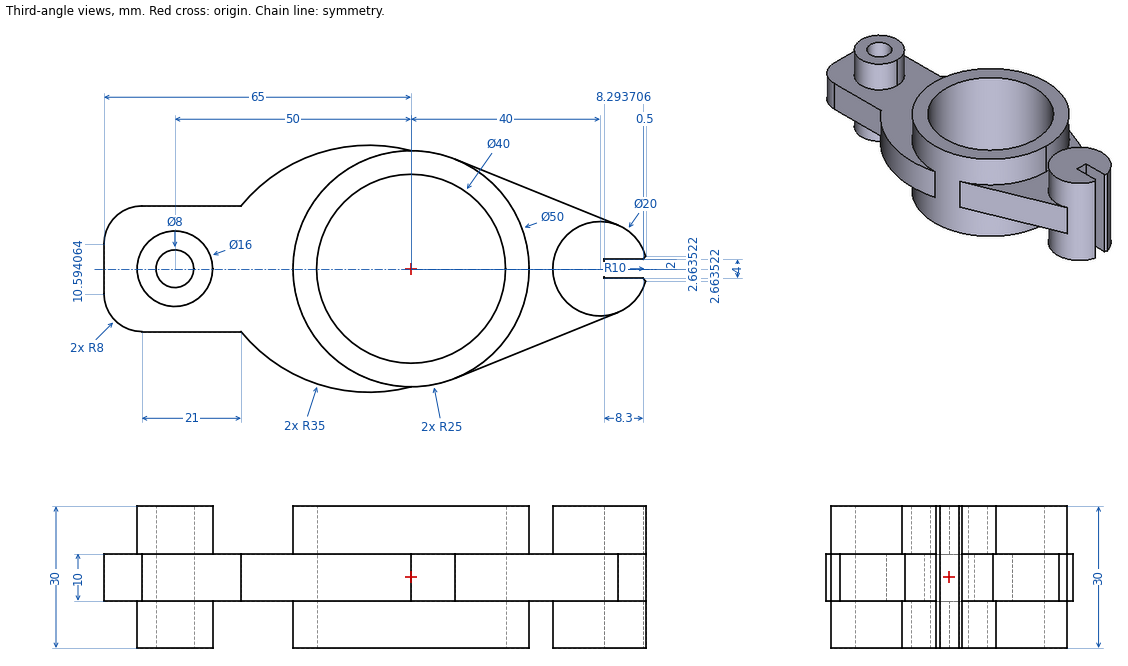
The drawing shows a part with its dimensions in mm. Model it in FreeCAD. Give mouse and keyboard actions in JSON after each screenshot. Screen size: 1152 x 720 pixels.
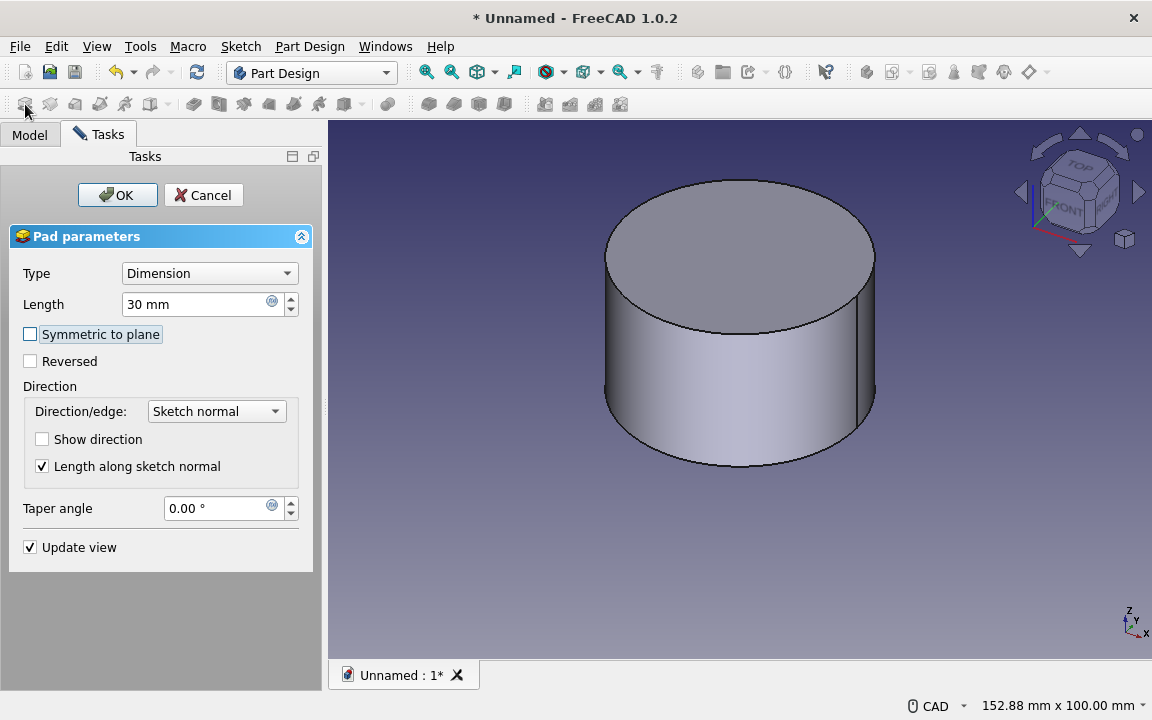
{"action": "left_click", "coordinate": [31, 334]}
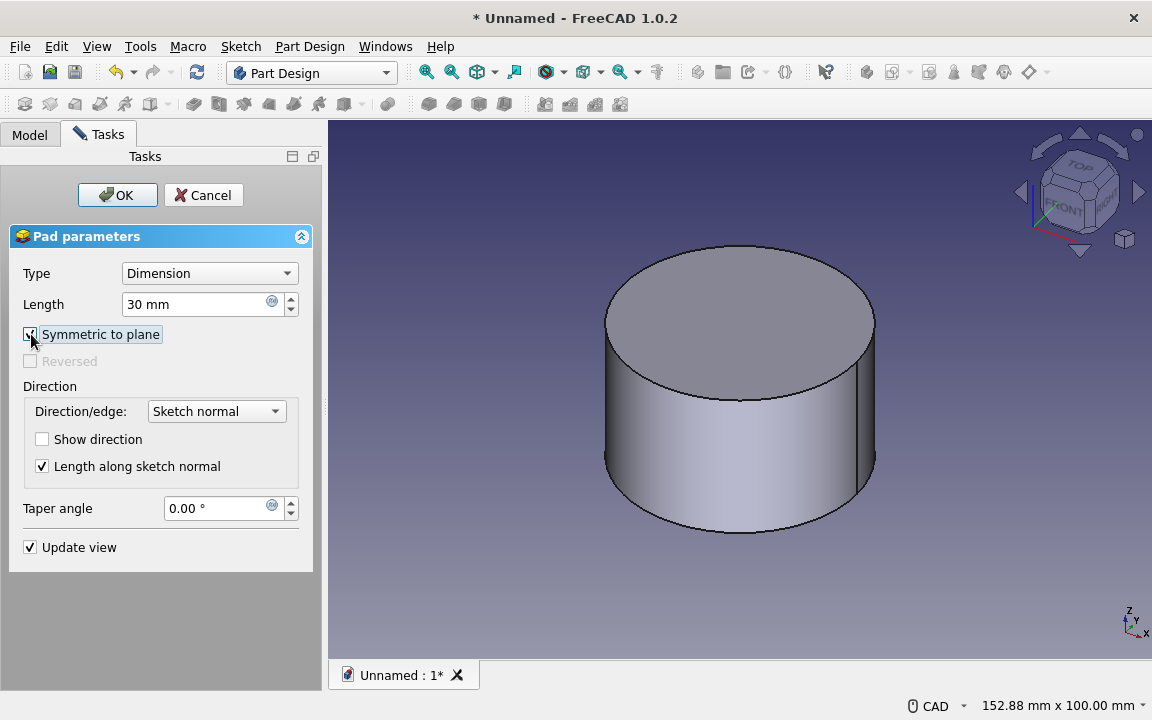
{"action": "left_click", "coordinate": [118, 195]}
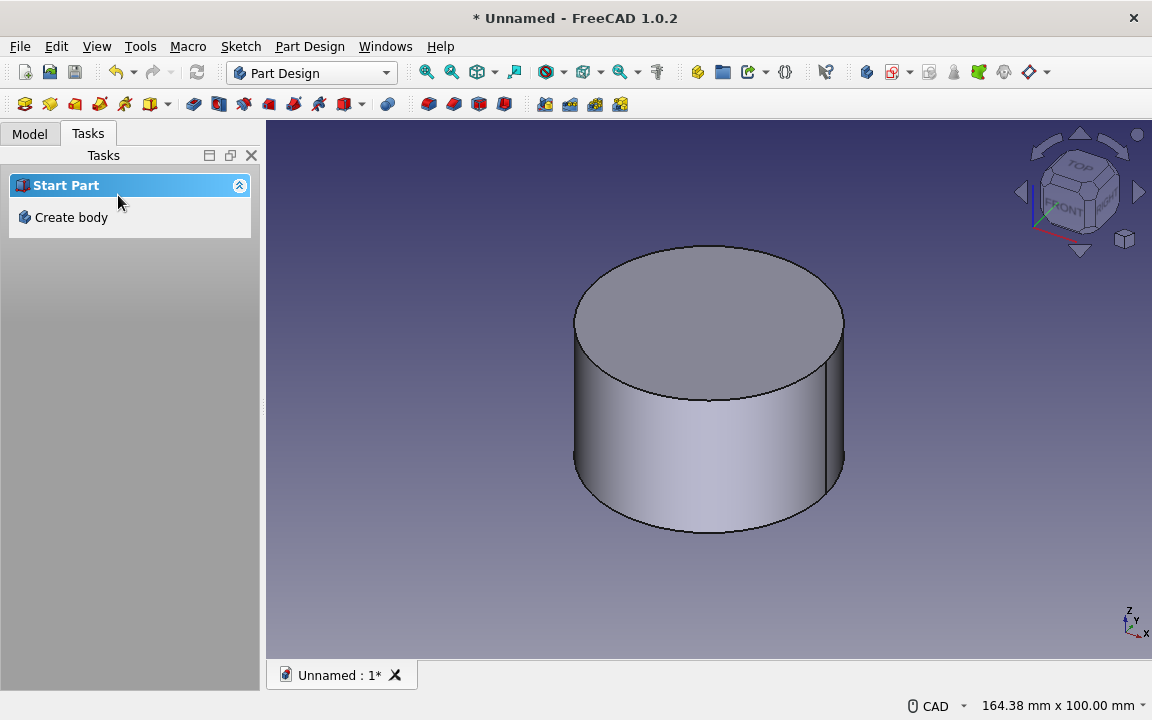
{"action": "left_click", "coordinate": [867, 72]}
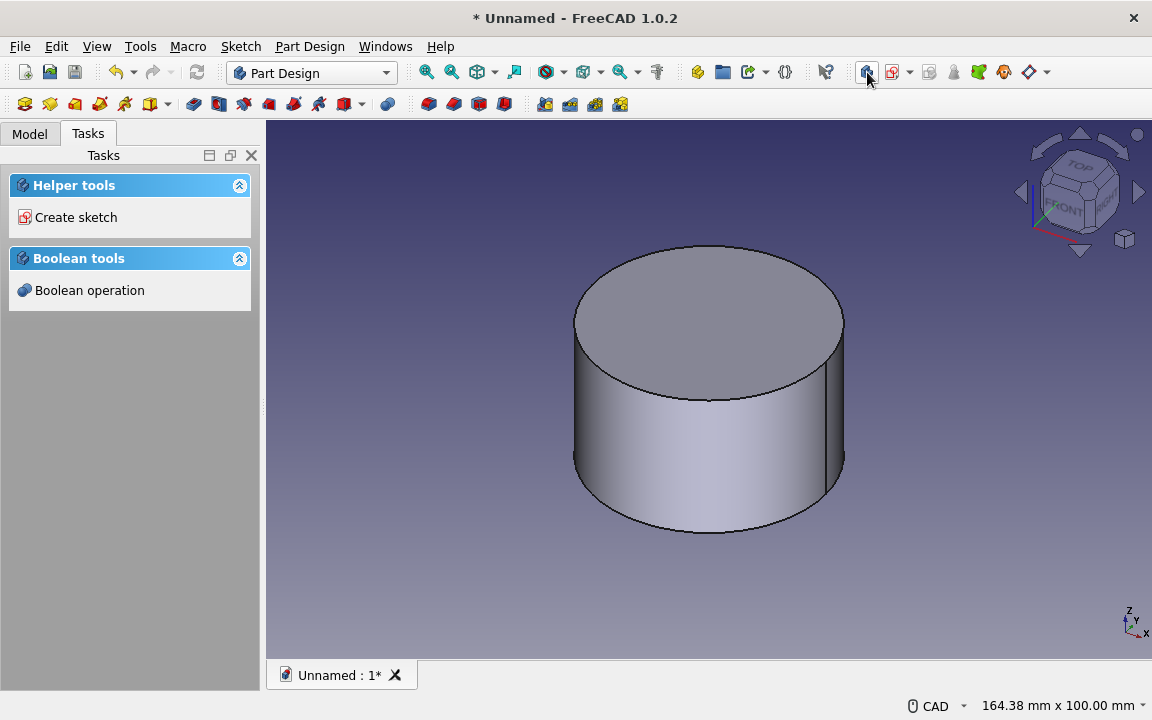
{"action": "left_click", "coordinate": [306, 619]}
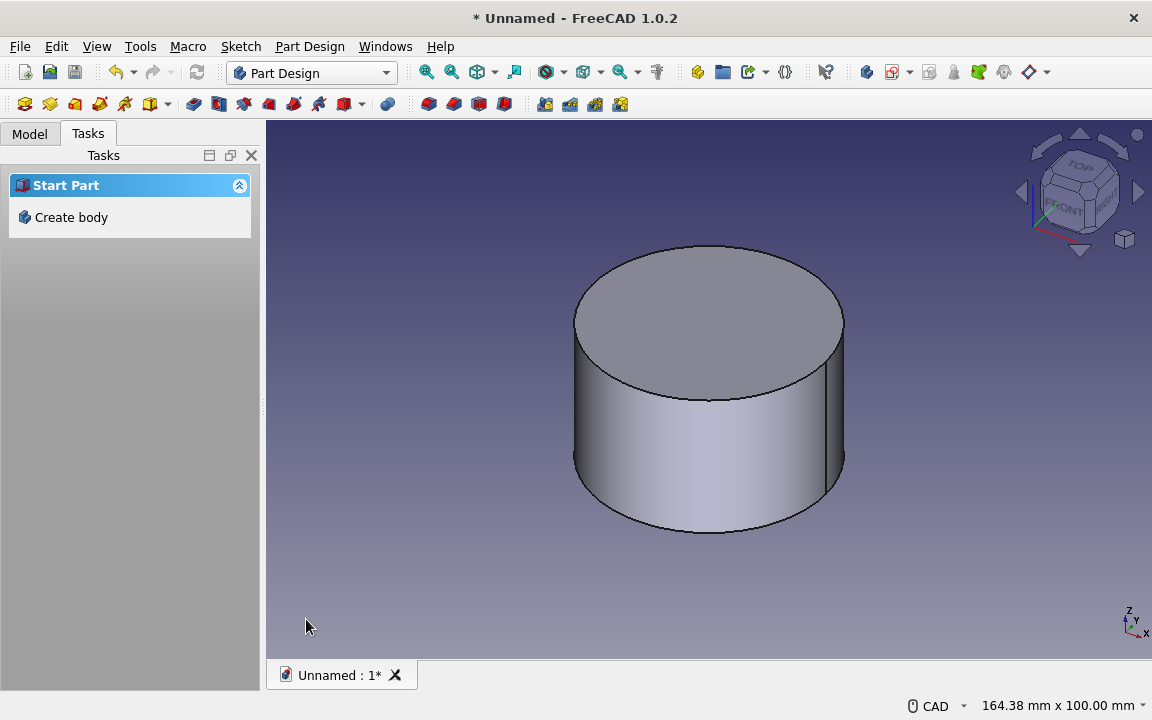
{"action": "left_click", "coordinate": [892, 72]}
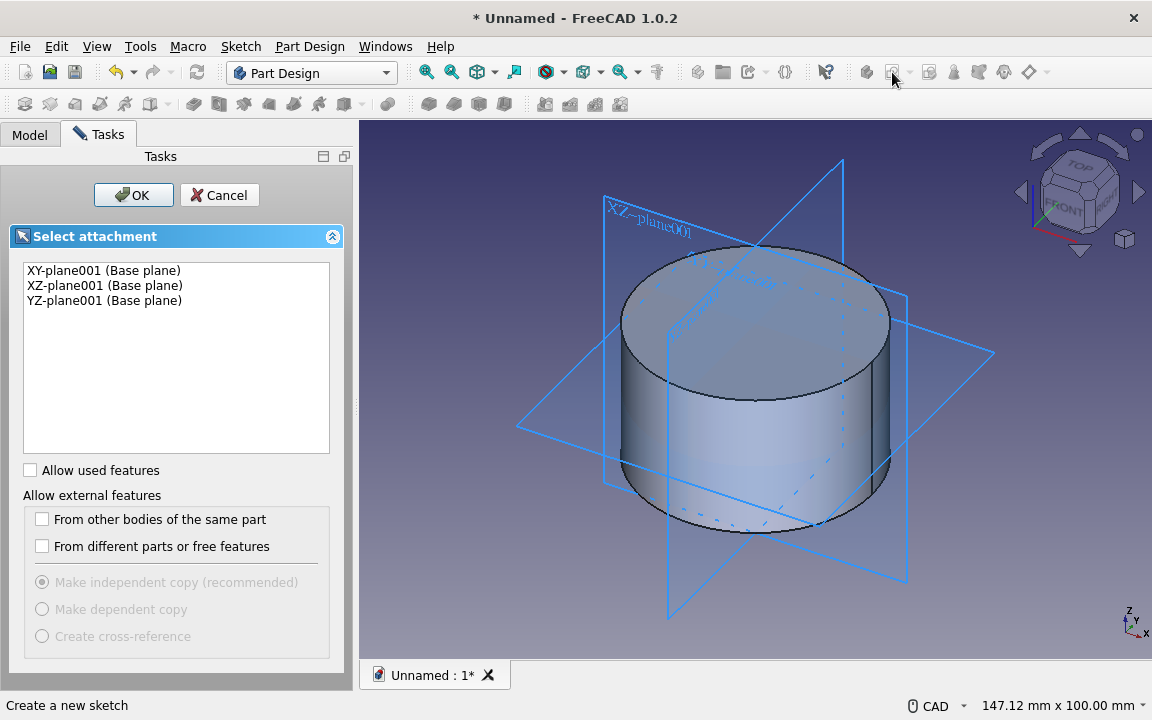
{"action": "left_click", "coordinate": [84, 270]}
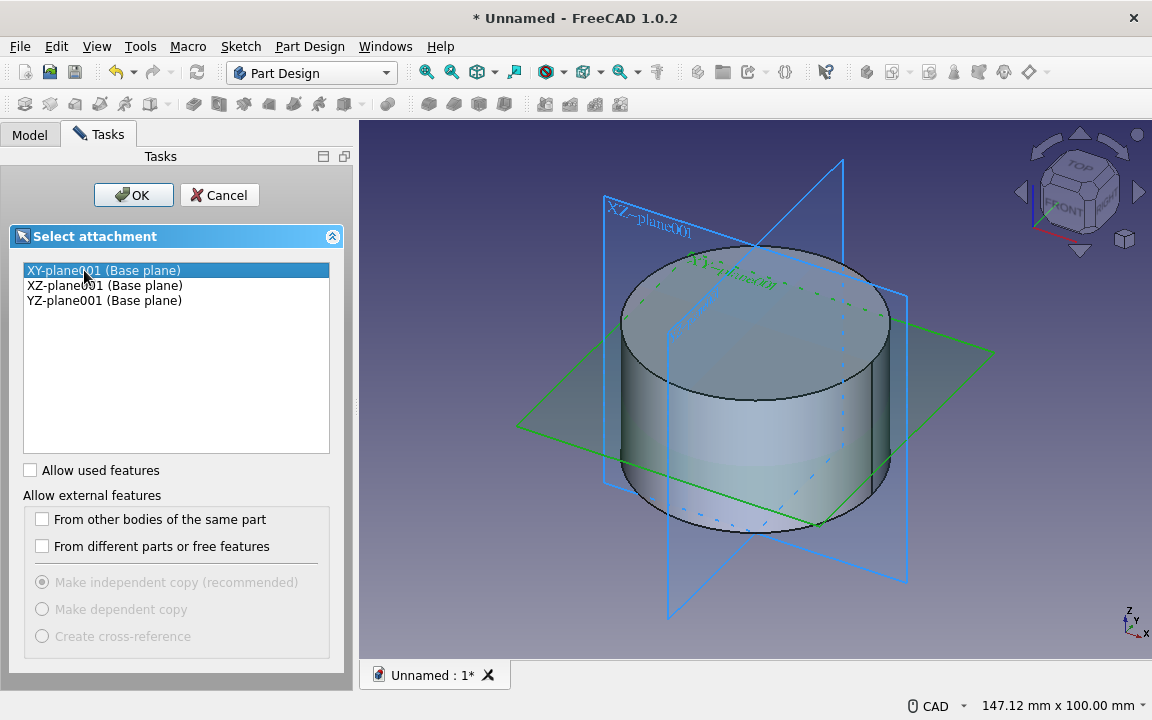
{"action": "left_click", "coordinate": [134, 195]}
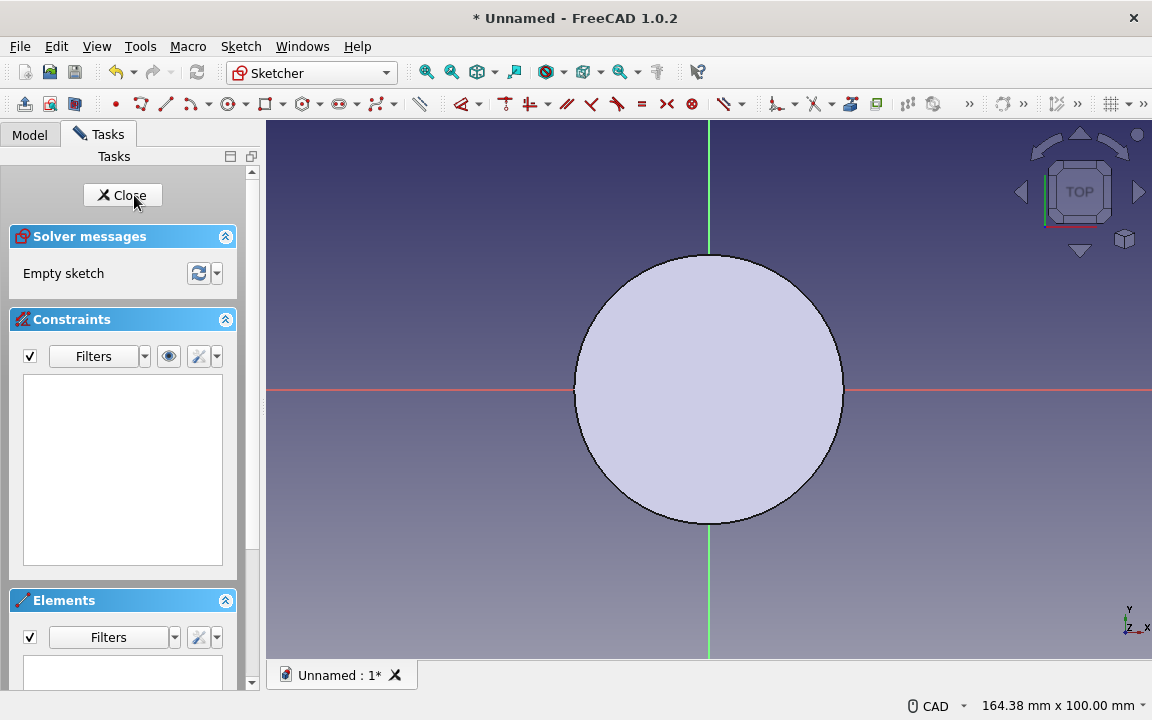
{"action": "scroll", "coordinate": [374, 390], "scroll_direction": "up", "scroll_amount": 7}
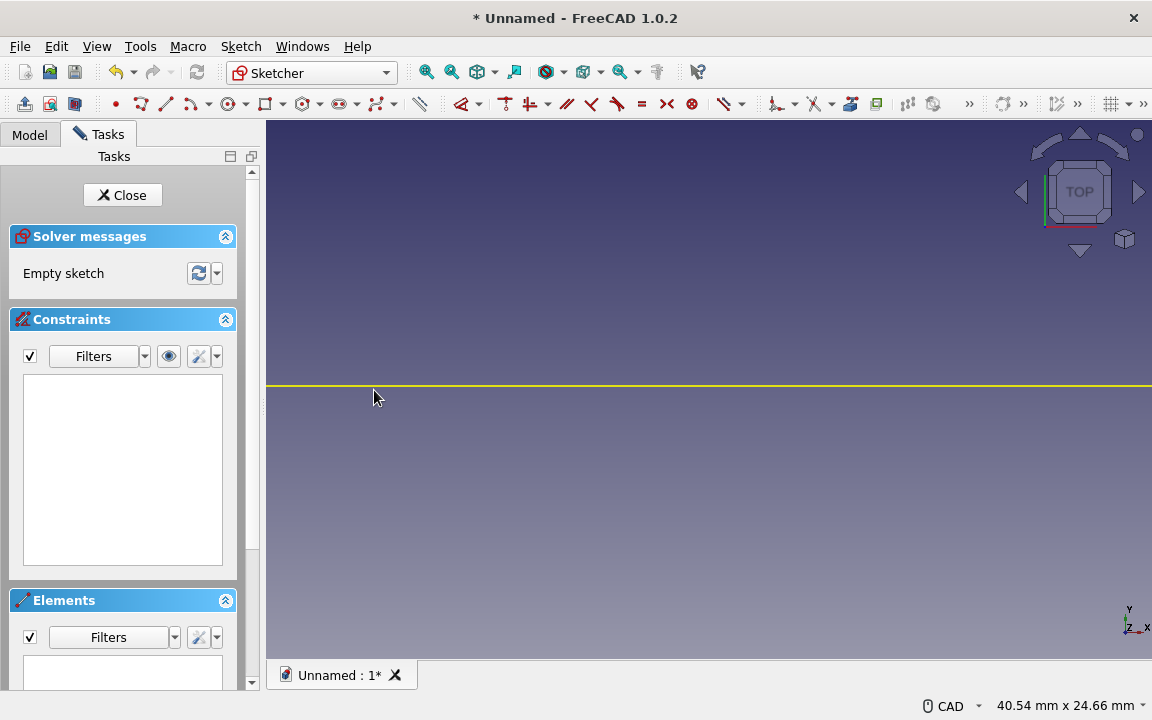
{"action": "left_click", "coordinate": [228, 104]}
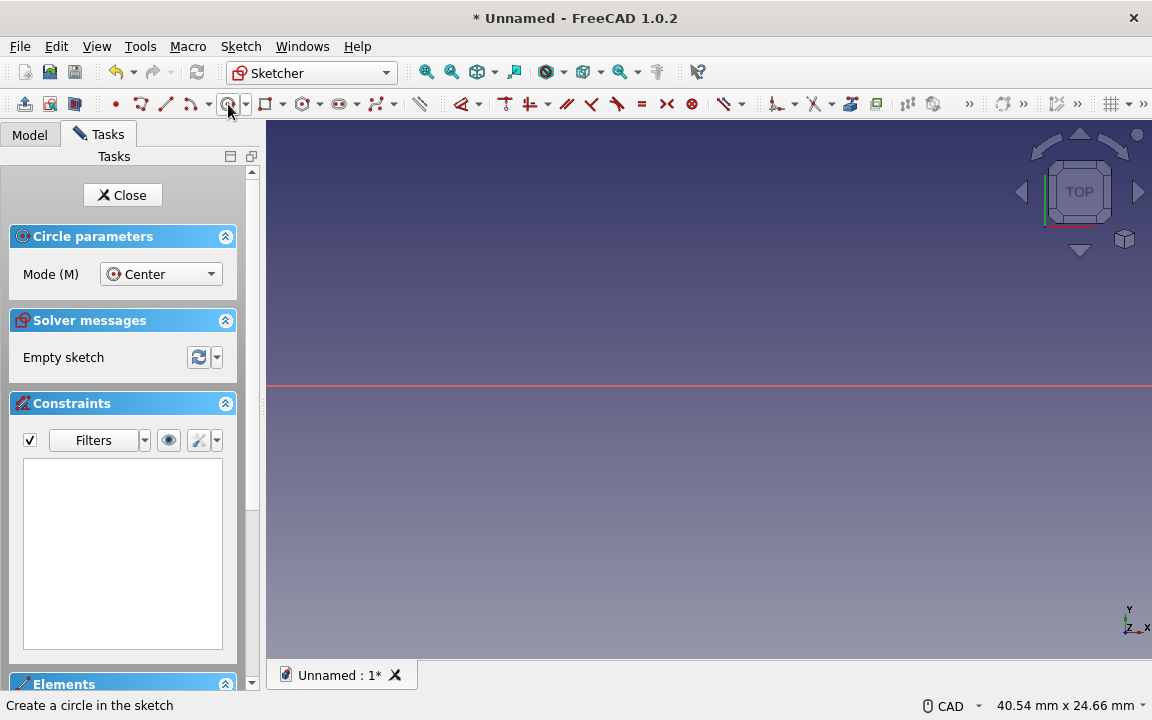
{"action": "left_click", "coordinate": [639, 386]}
{"action": "left_click", "coordinate": [763, 263]}
{"action": "key", "text": "Escape"}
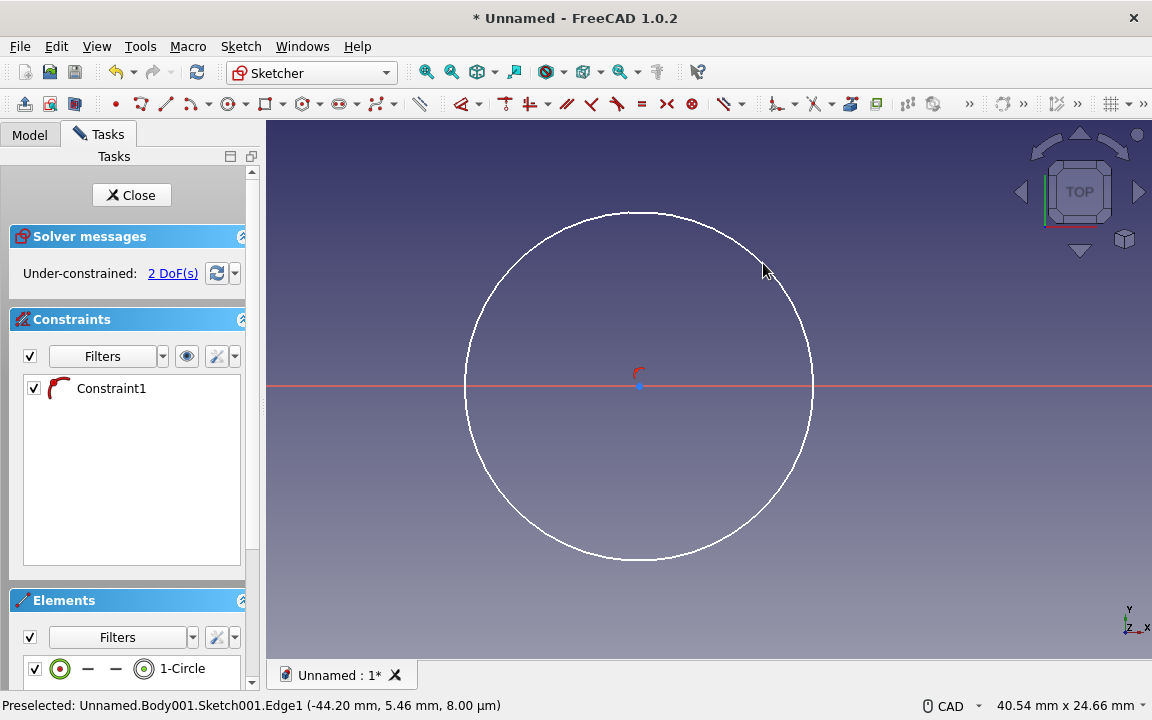
{"action": "left_click", "coordinate": [460, 104]}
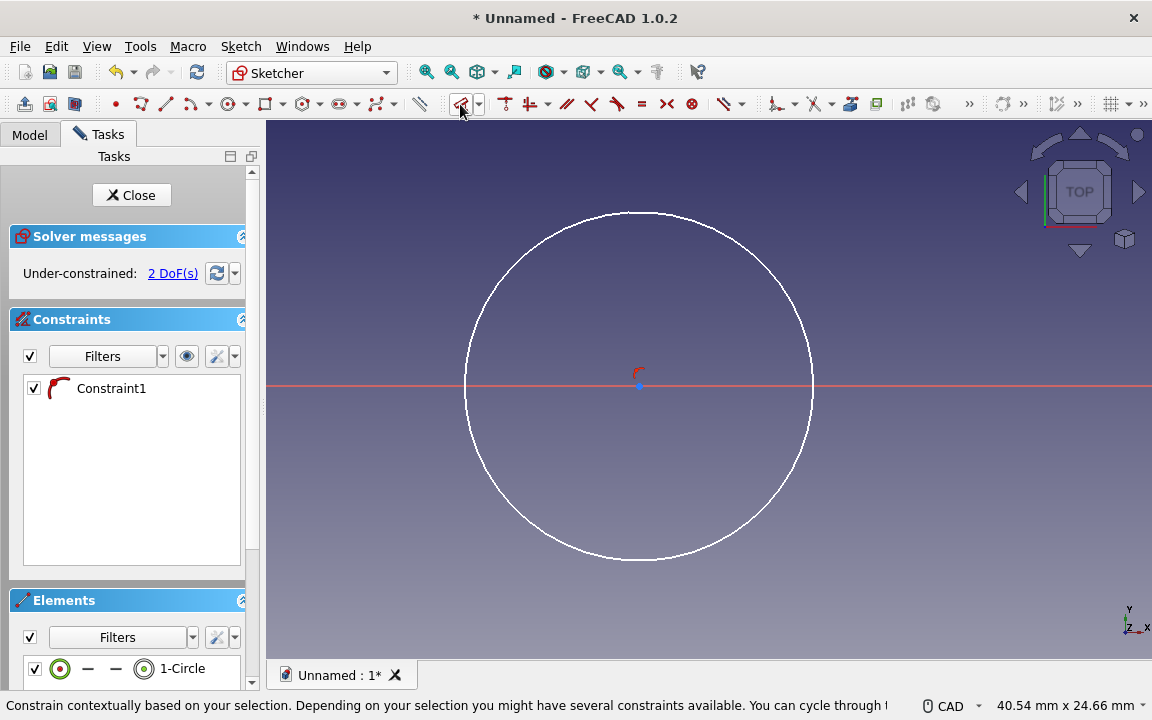
{"action": "left_click", "coordinate": [762, 263]}
{"action": "left_click", "coordinate": [785, 240]}